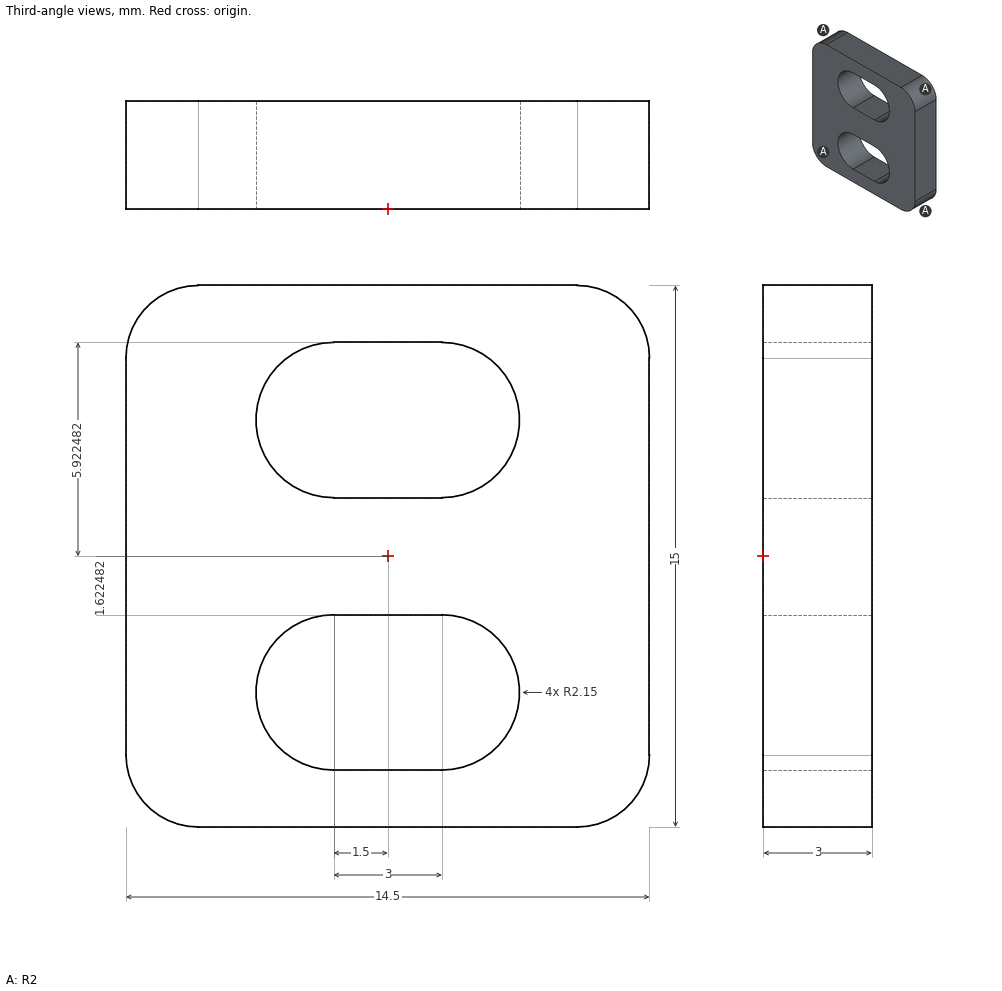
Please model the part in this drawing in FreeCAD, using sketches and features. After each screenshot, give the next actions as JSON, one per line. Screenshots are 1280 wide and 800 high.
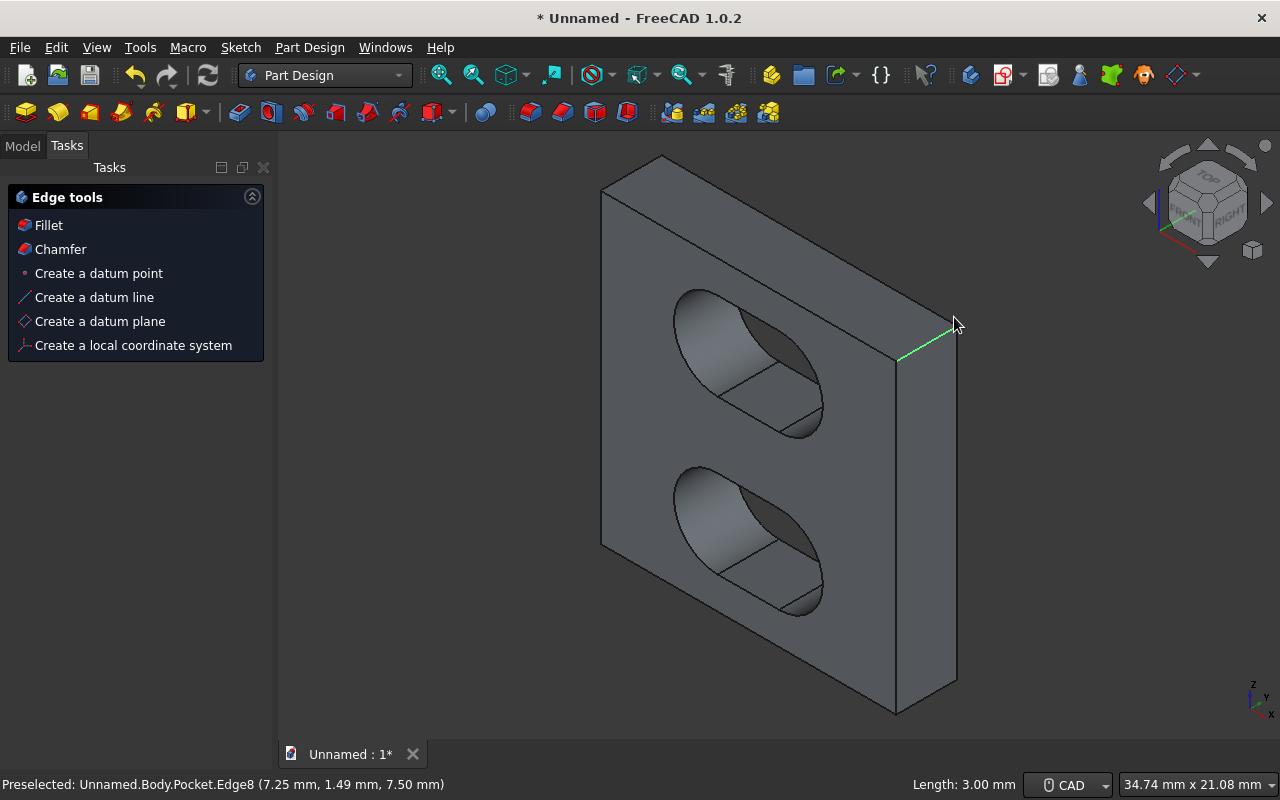
{"action": "key", "text": "2"}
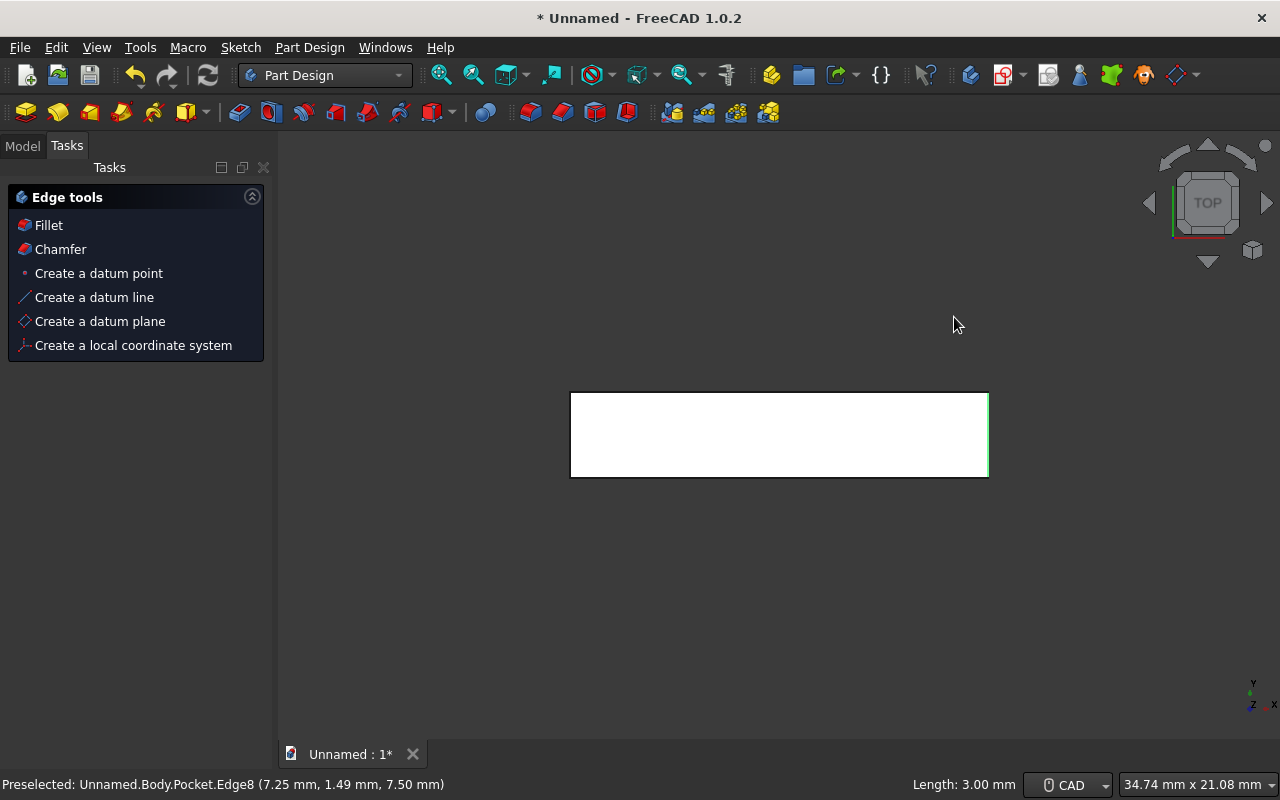
{"action": "left_click", "coordinate": [442, 76]}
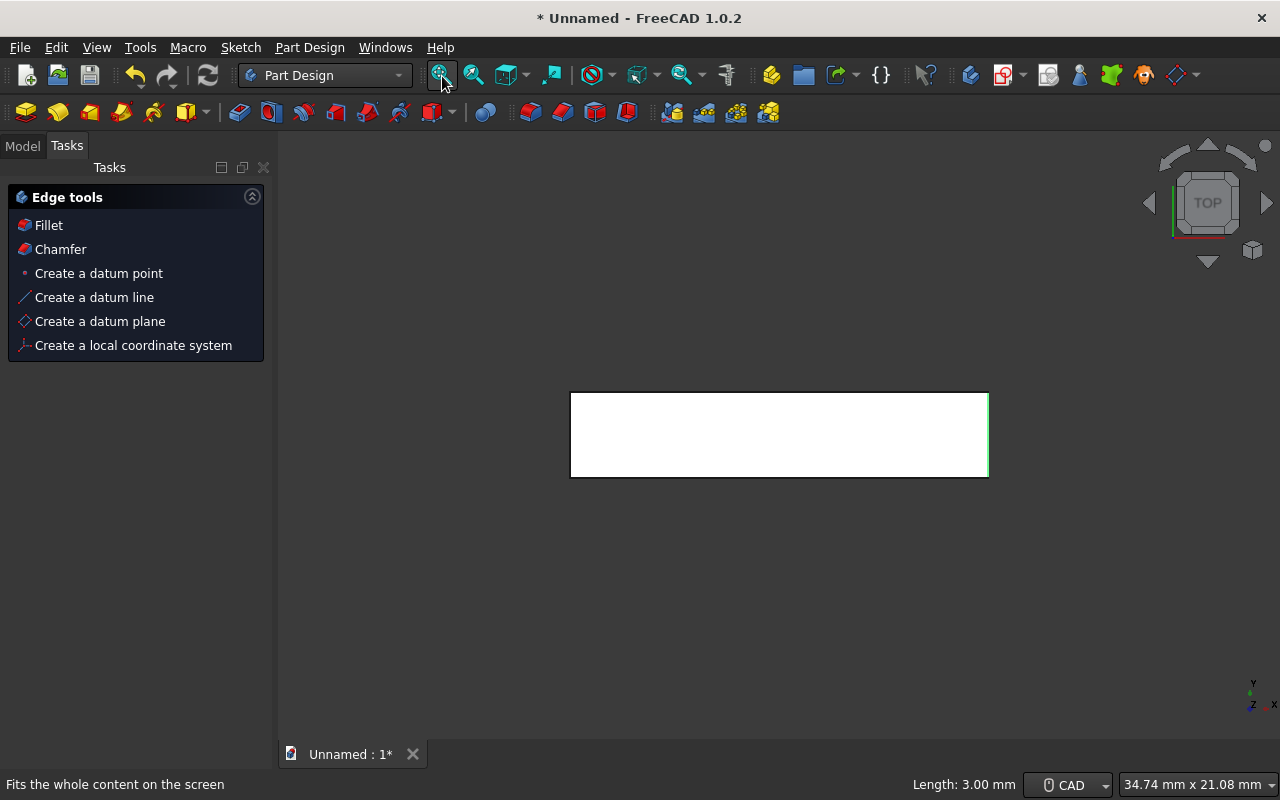
{"action": "left_click", "coordinate": [570, 434], "text": "ctrl"}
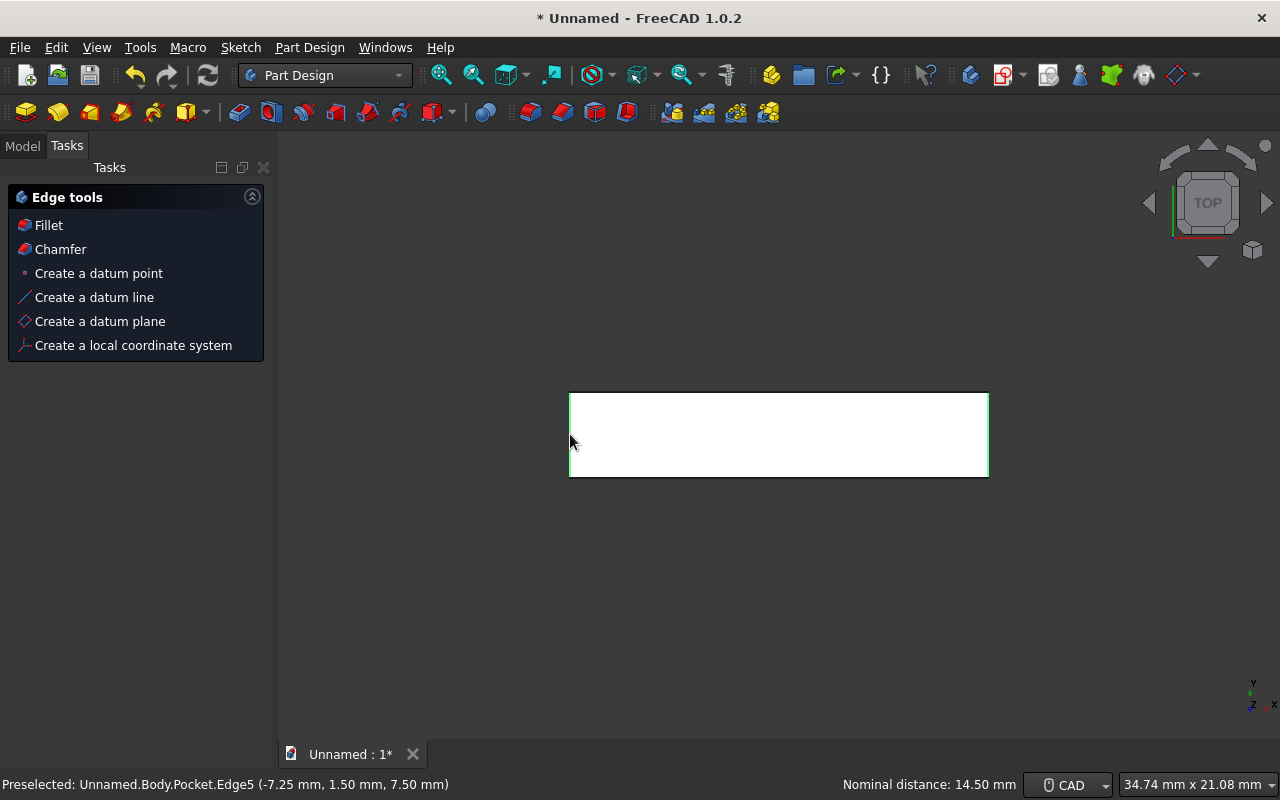
{"action": "key", "text": "1"}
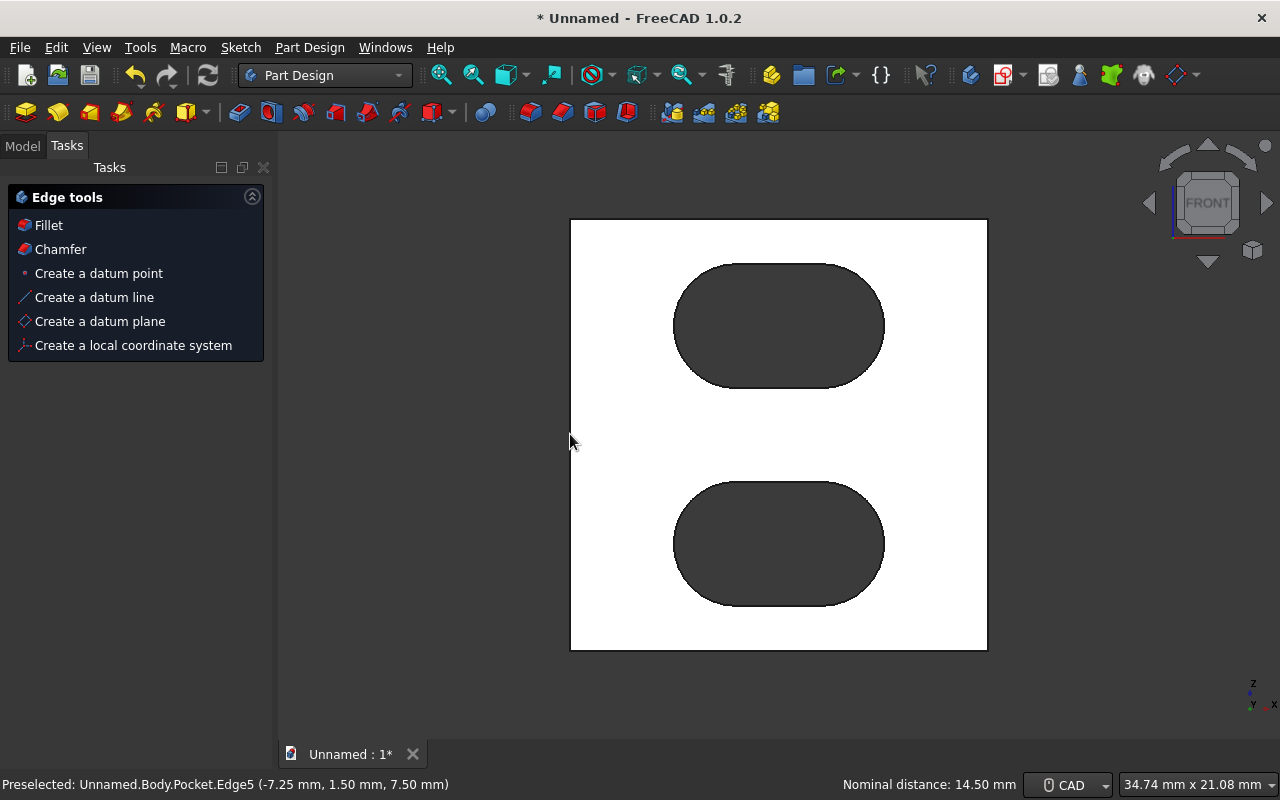
{"action": "key", "text": "3"}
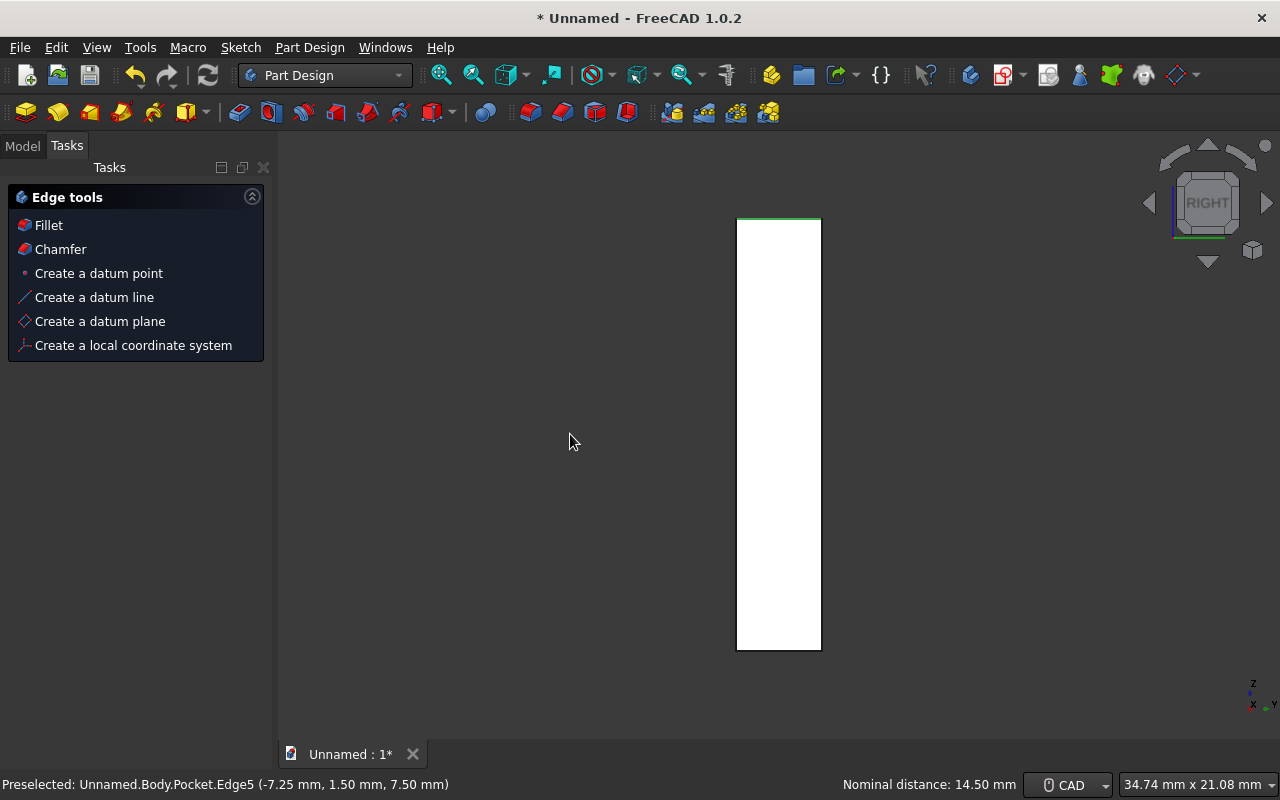
{"action": "left_click", "coordinate": [779, 650], "text": "ctrl"}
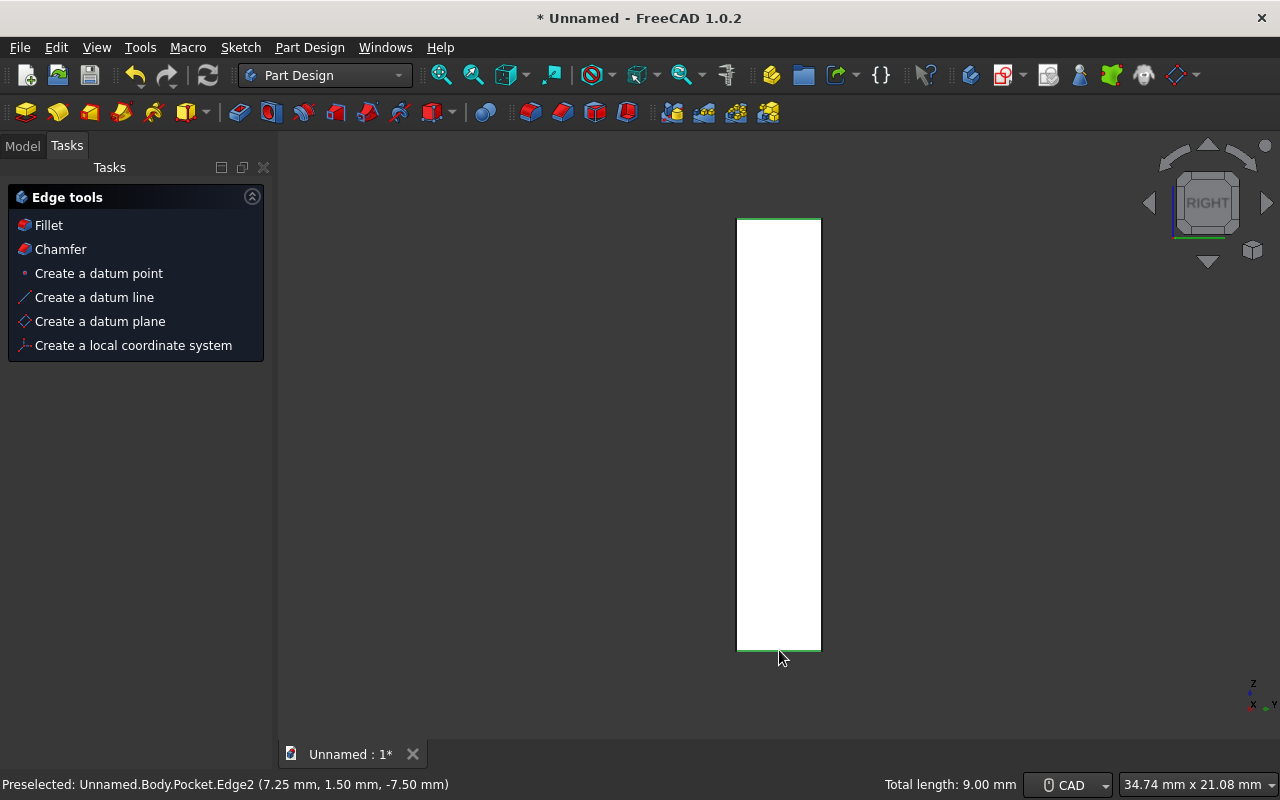
{"action": "key", "text": "5"}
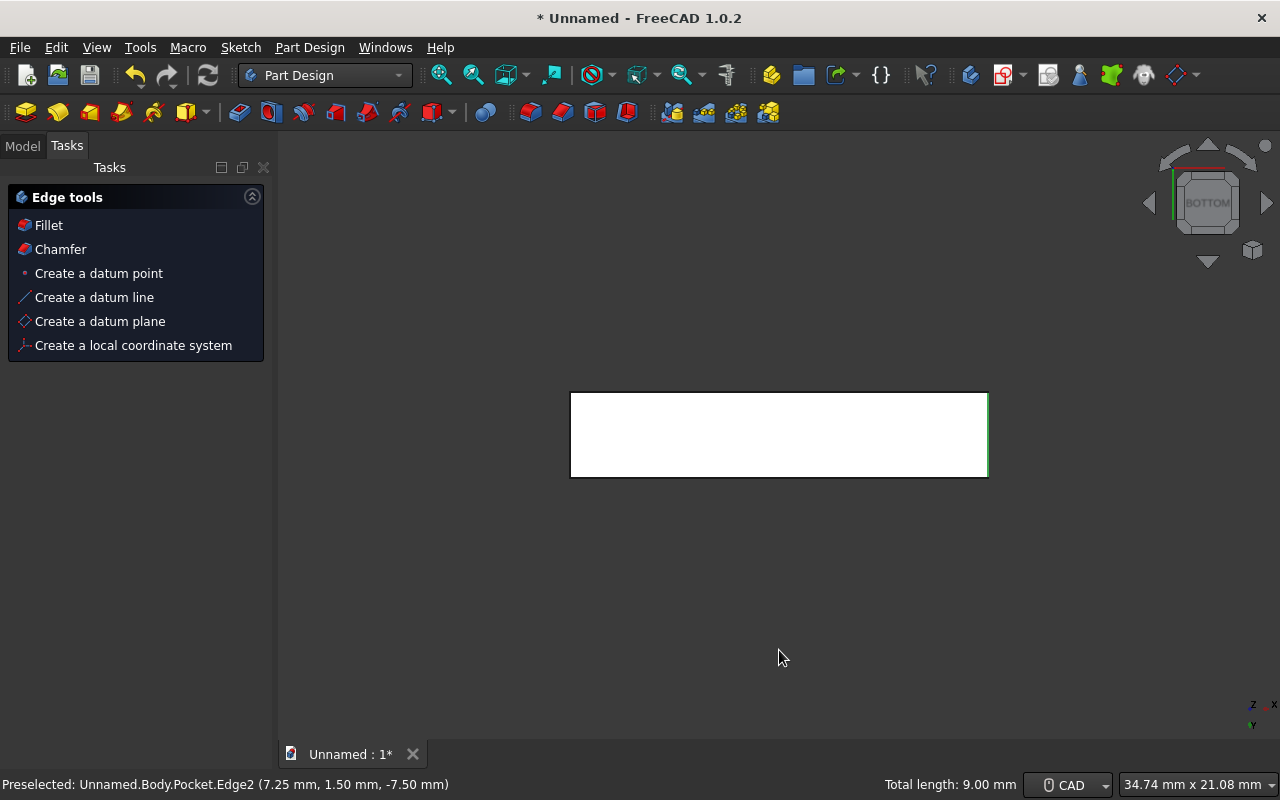
{"action": "left_click", "coordinate": [442, 76]}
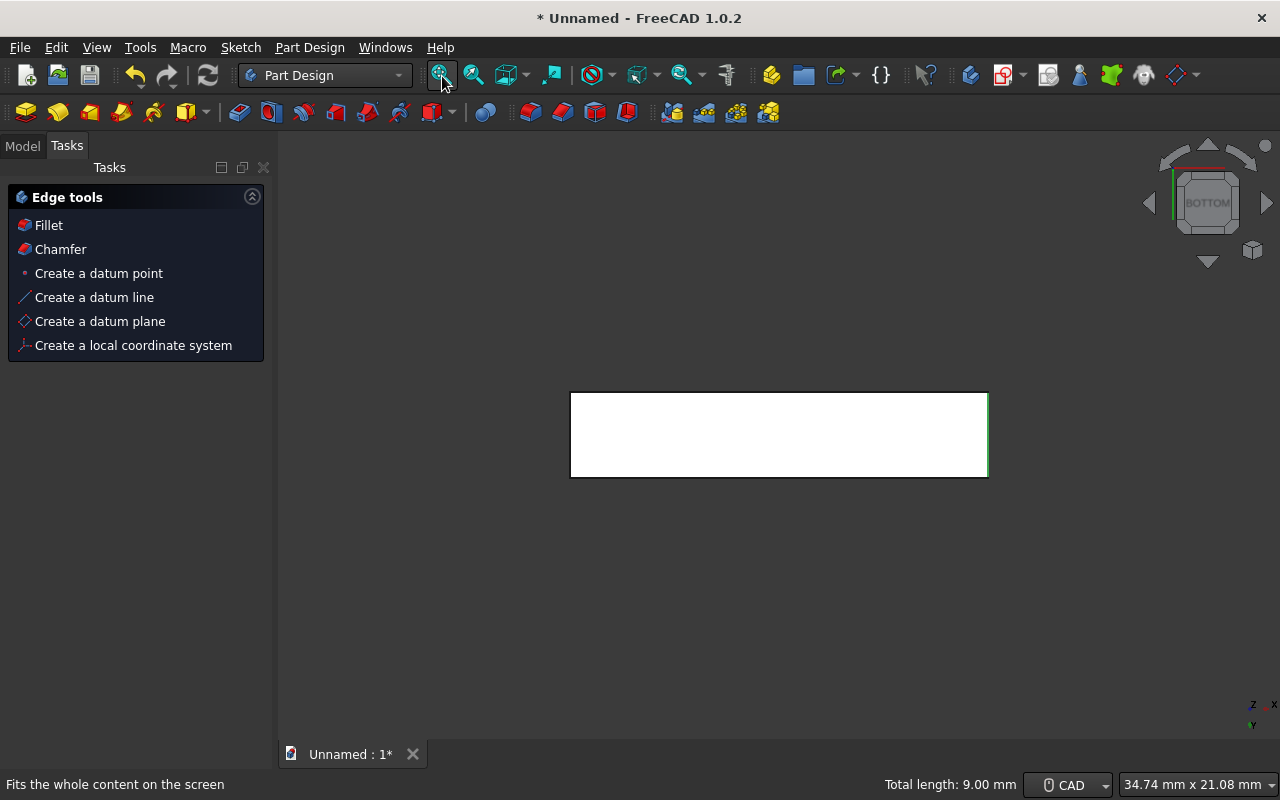
{"action": "left_click", "coordinate": [570, 434], "text": "ctrl"}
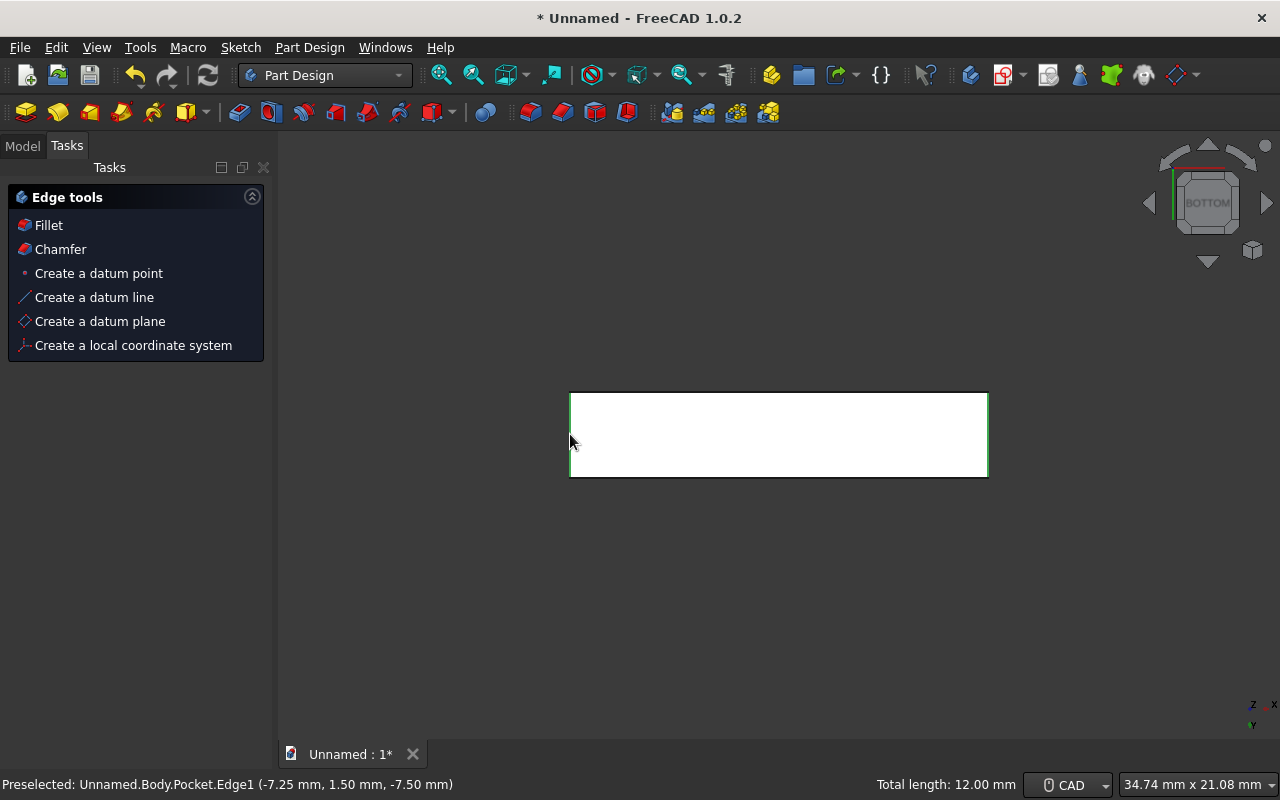
{"action": "left_click", "coordinate": [532, 112]}